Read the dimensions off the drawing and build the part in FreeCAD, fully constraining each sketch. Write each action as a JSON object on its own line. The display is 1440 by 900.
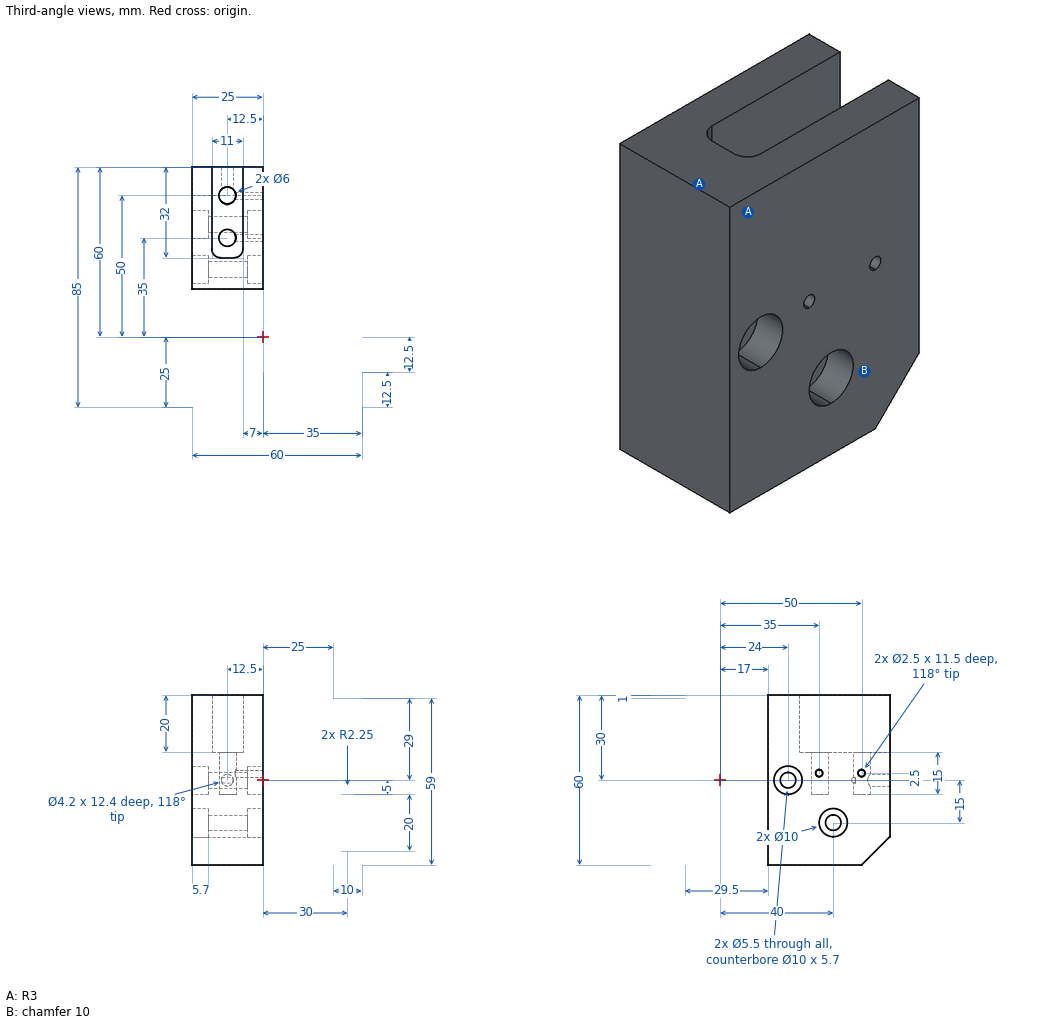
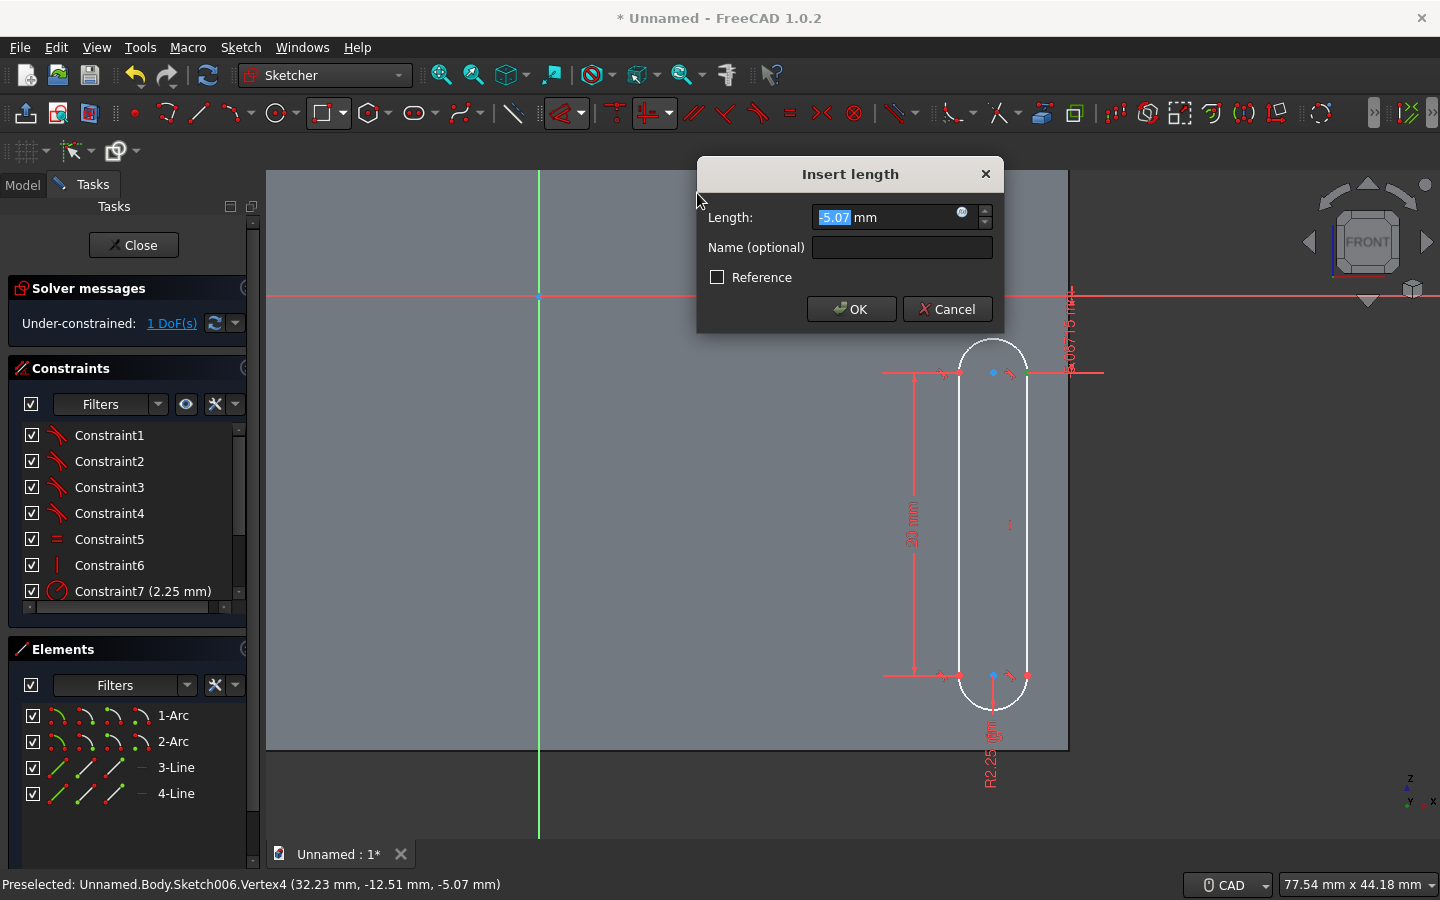
{"action": "type", "text": "-5"}
{"action": "key", "text": "Return"}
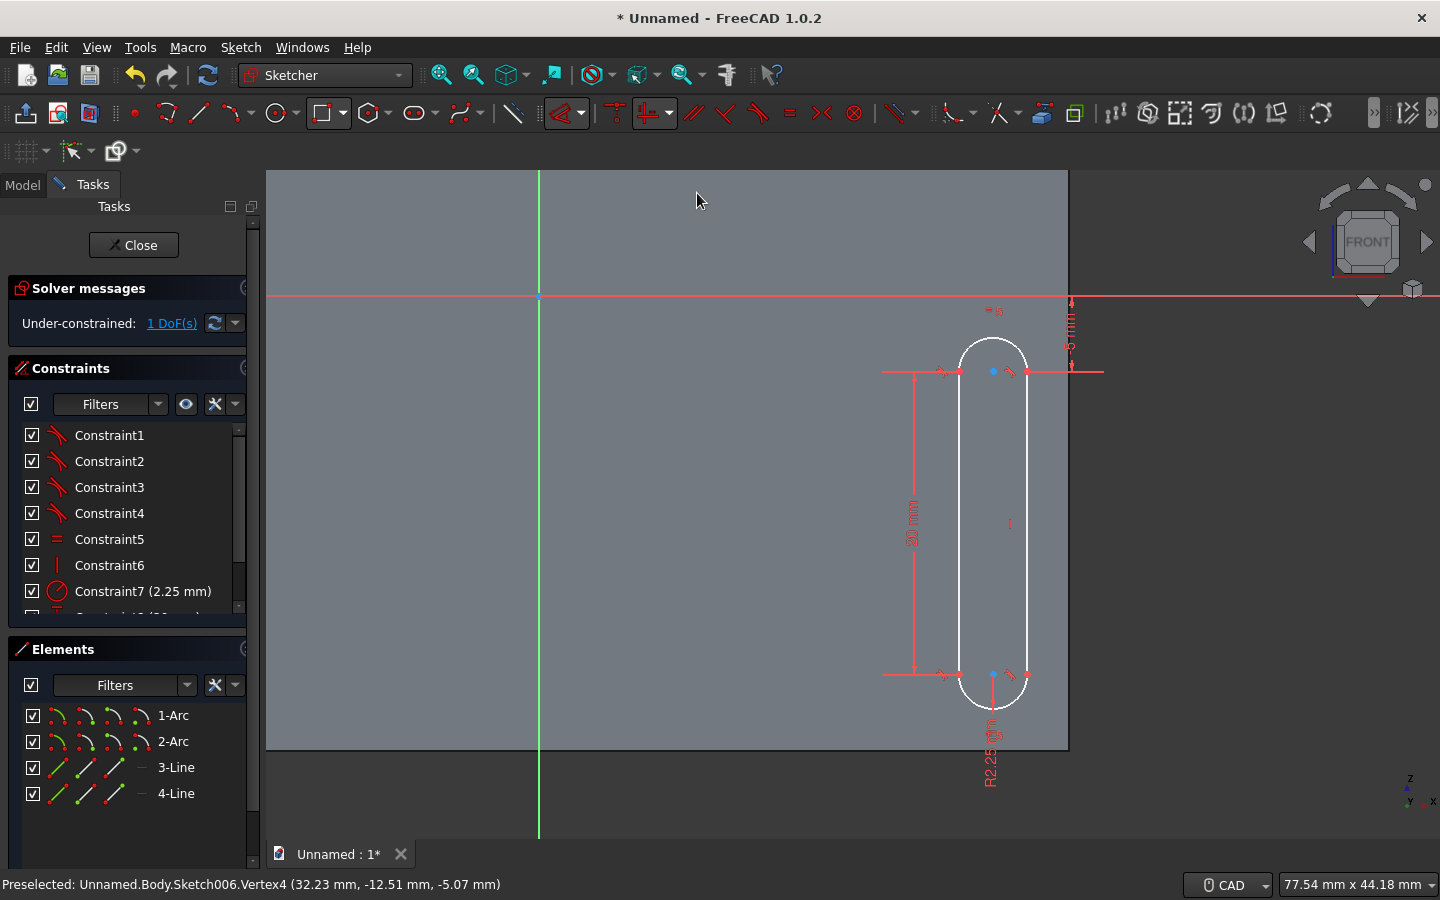
{"action": "left_click", "coordinate": [993, 675]}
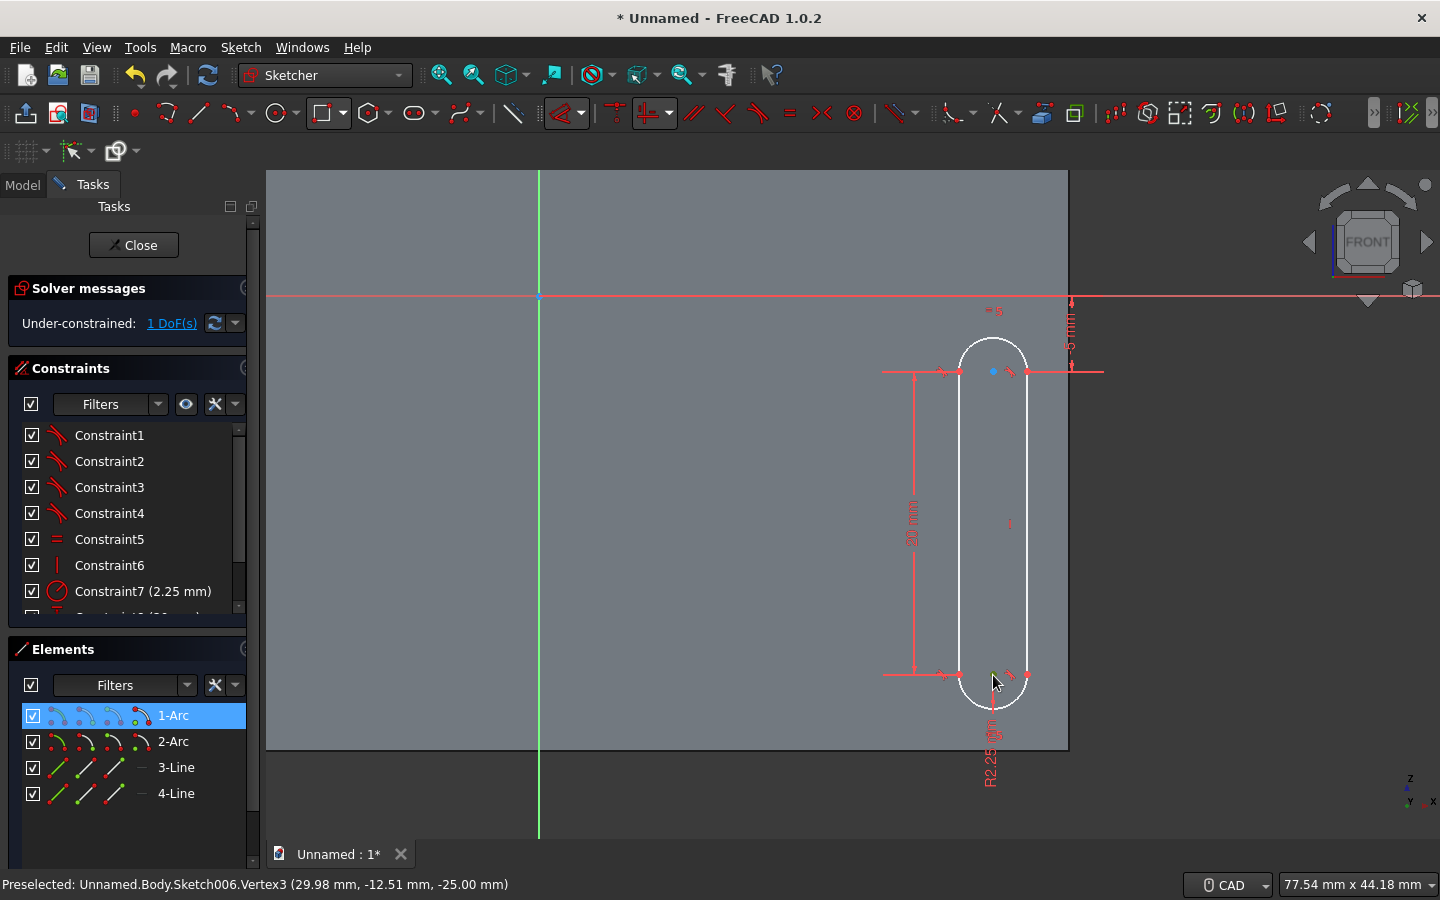
{"action": "key", "text": "l"}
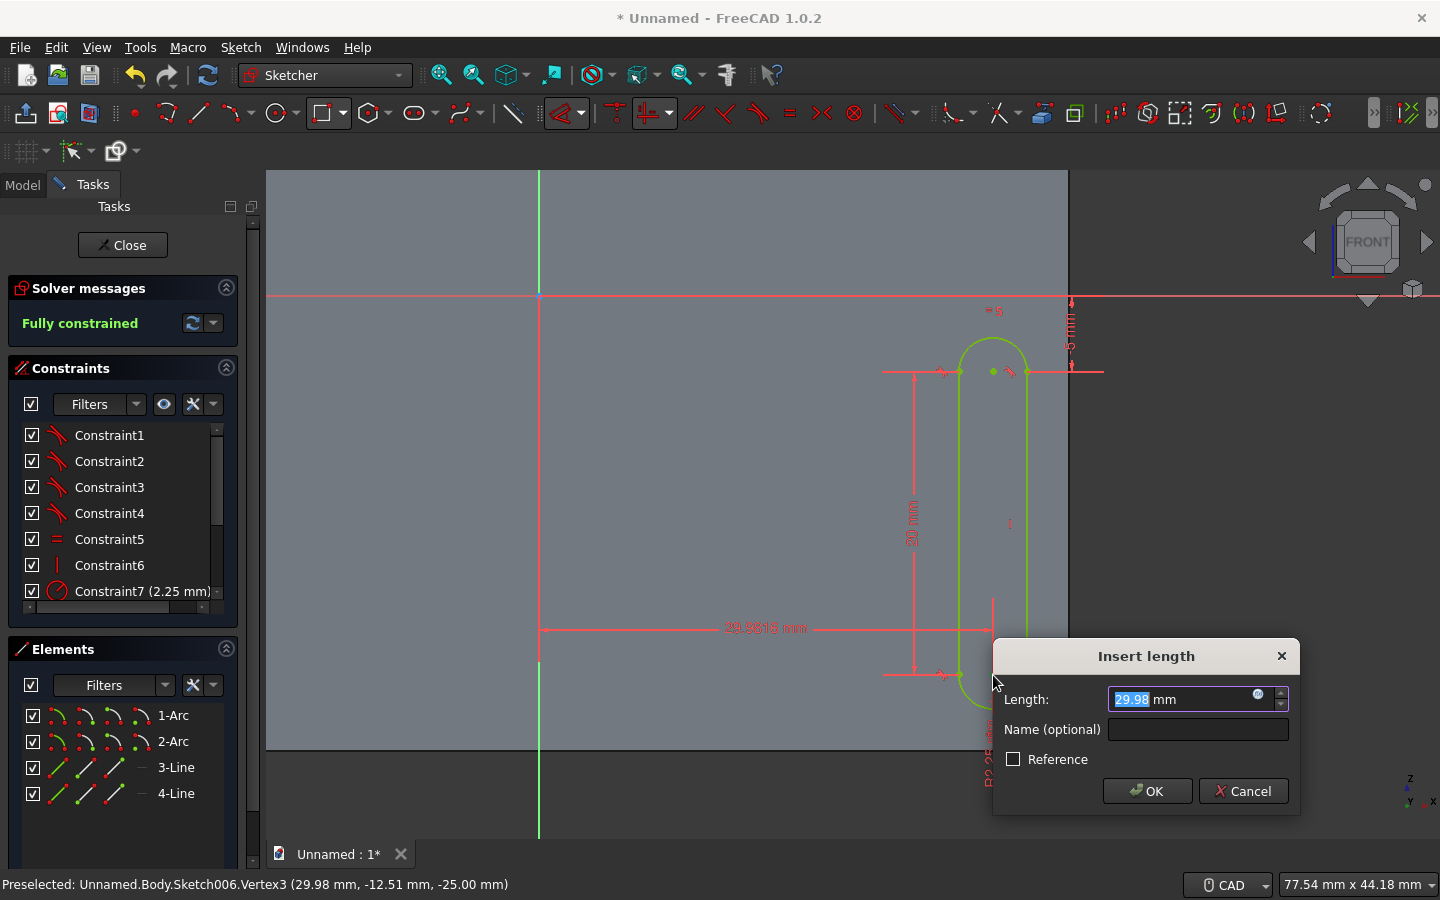
{"action": "type", "text": "30"}
{"action": "key", "text": "Return"}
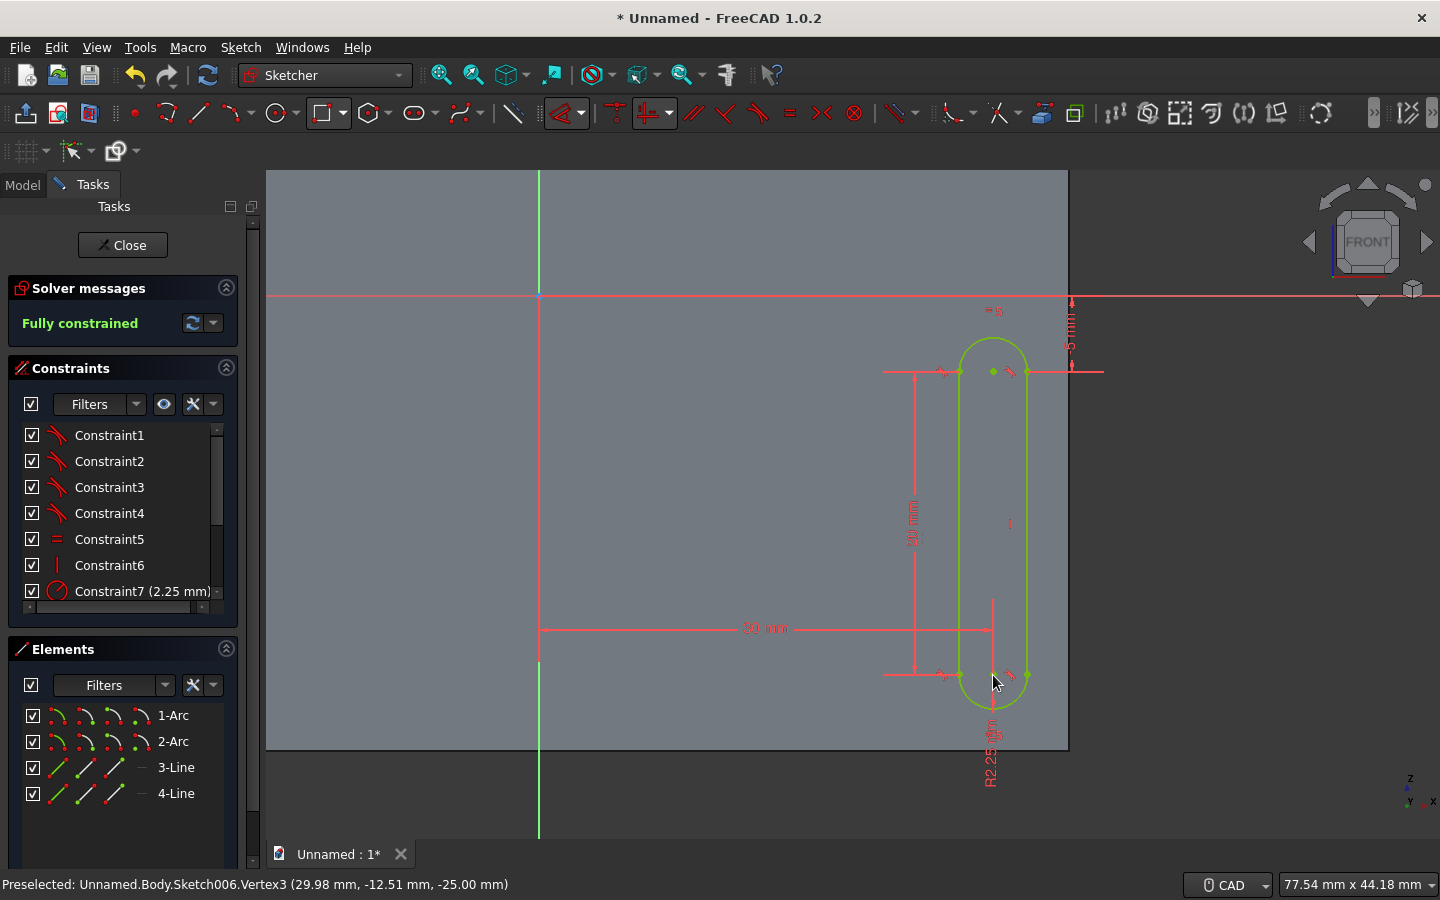
{"action": "left_click", "coordinate": [123, 245]}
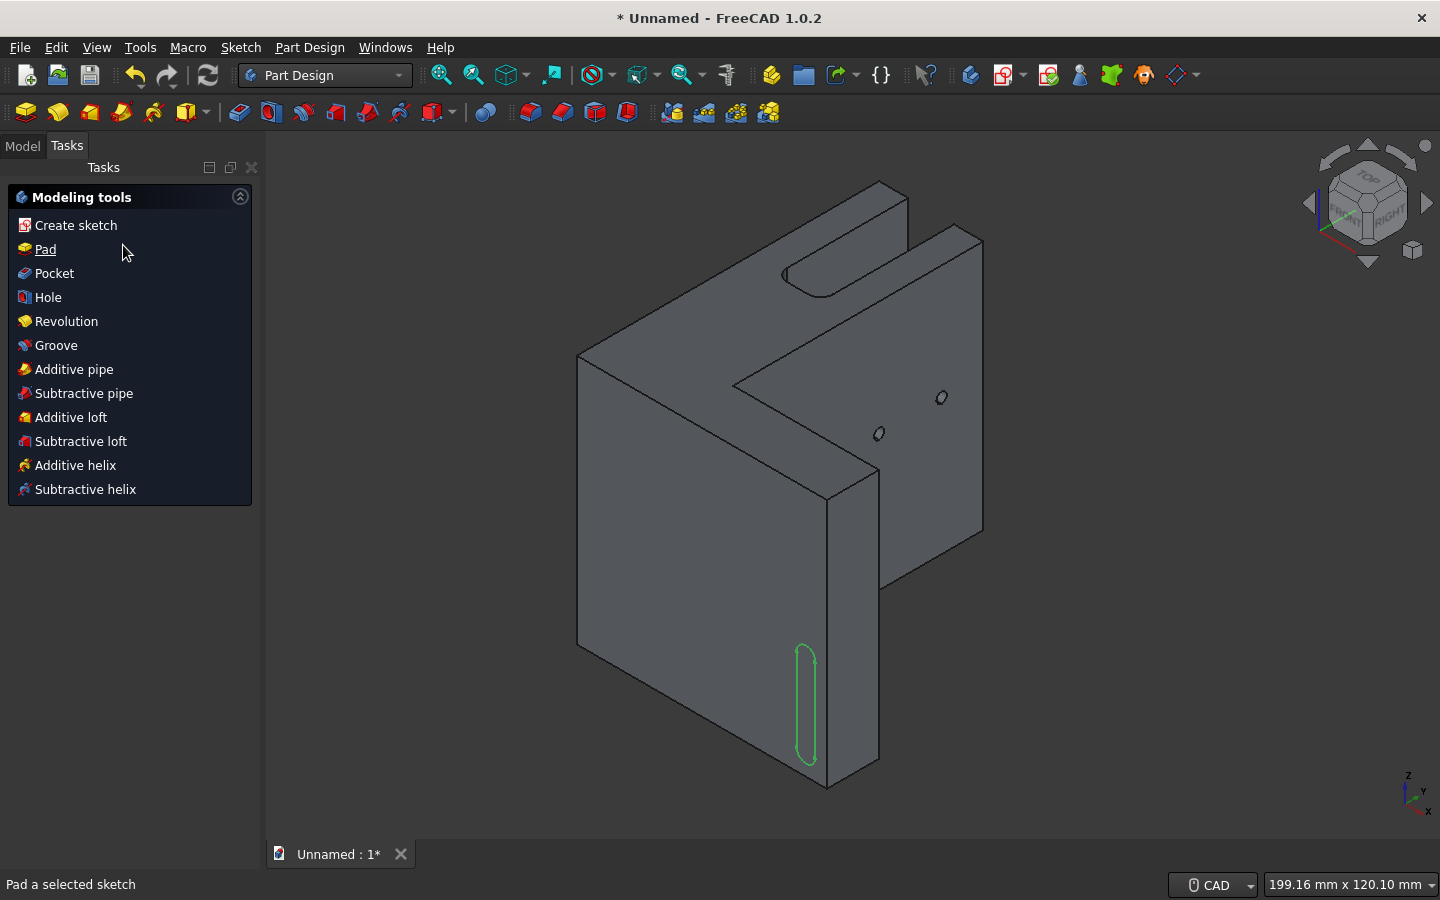
{"action": "left_click", "coordinate": [240, 112]}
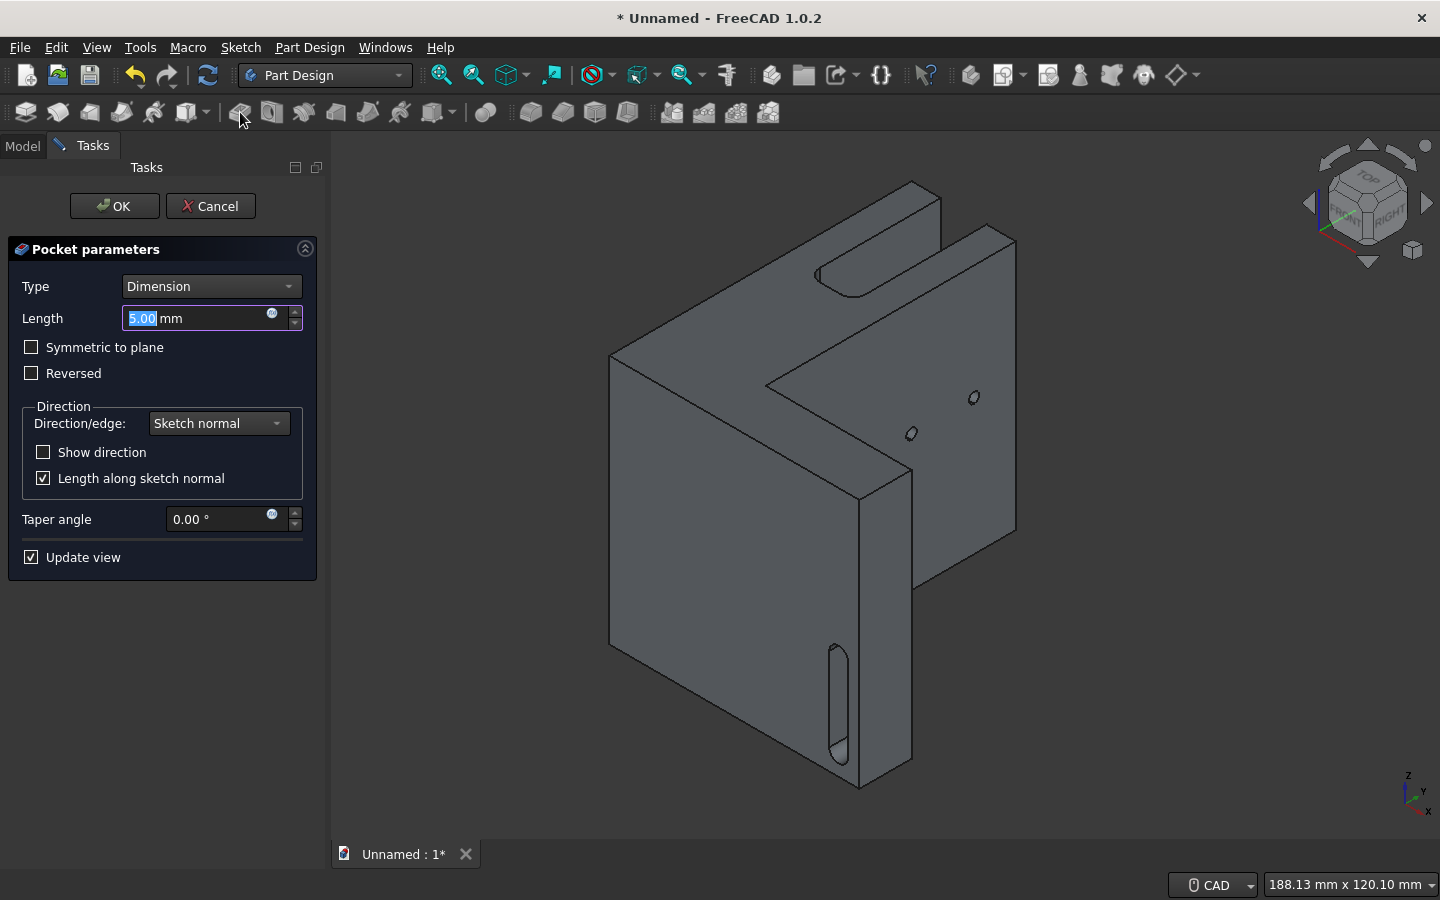
{"action": "left_click", "coordinate": [212, 286]}